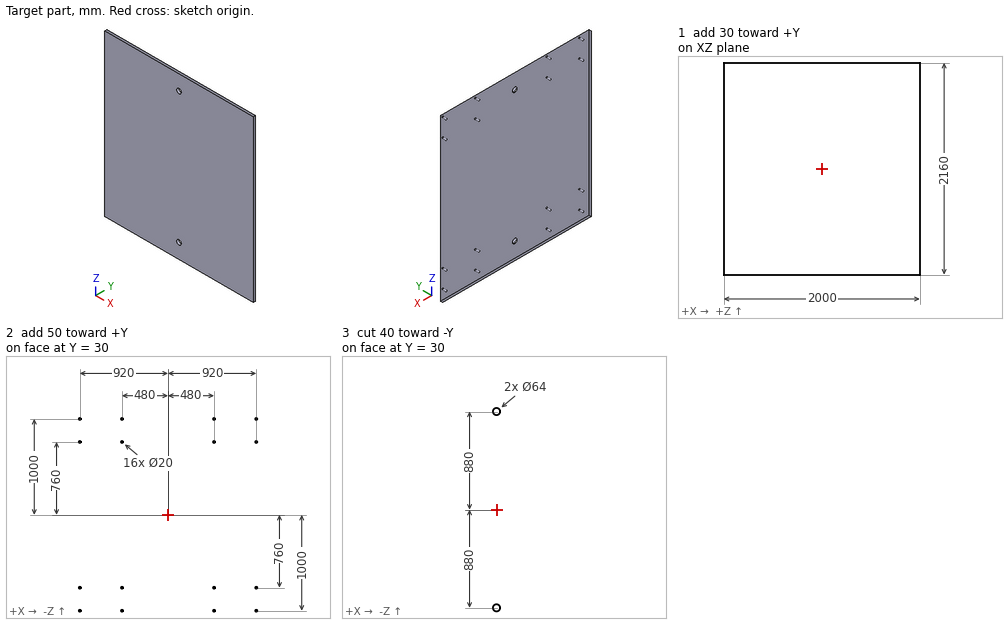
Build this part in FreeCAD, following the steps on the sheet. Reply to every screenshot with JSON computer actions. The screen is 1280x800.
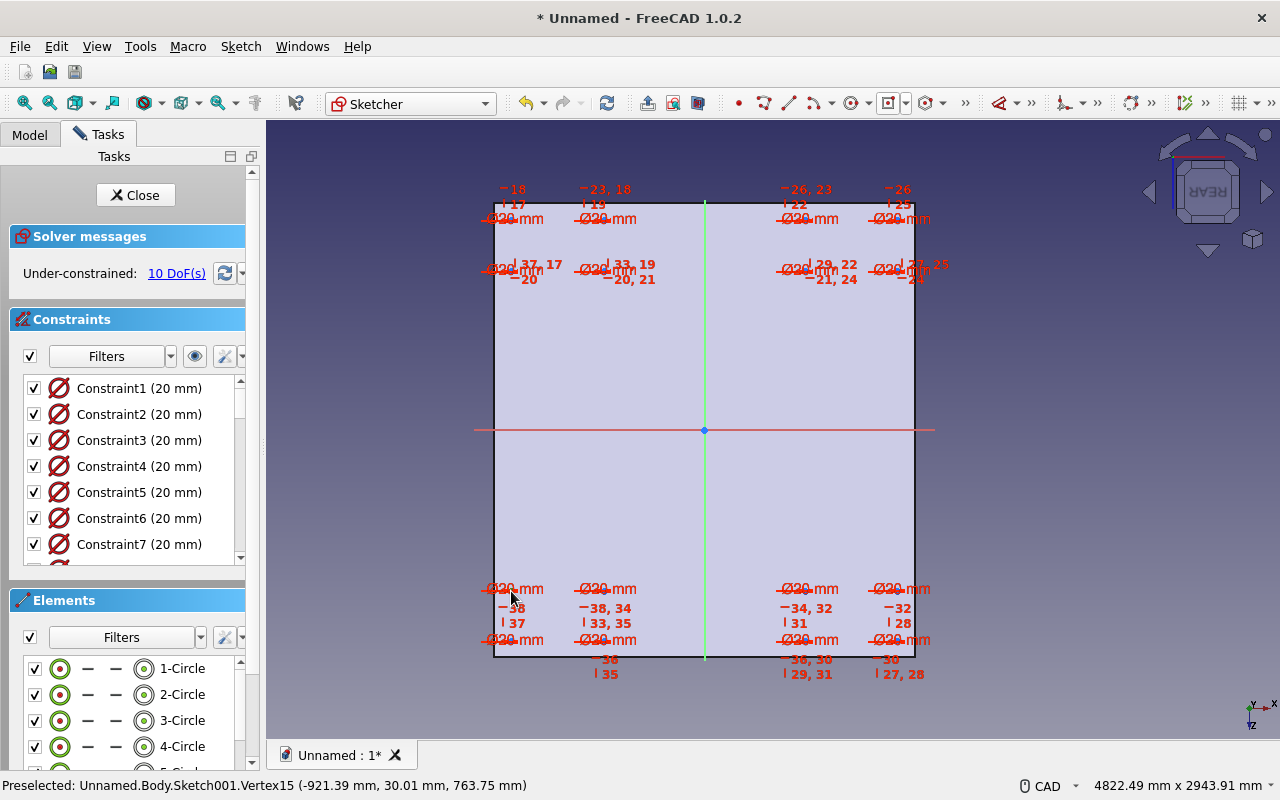
{"action": "left_click", "coordinate": [511, 642]}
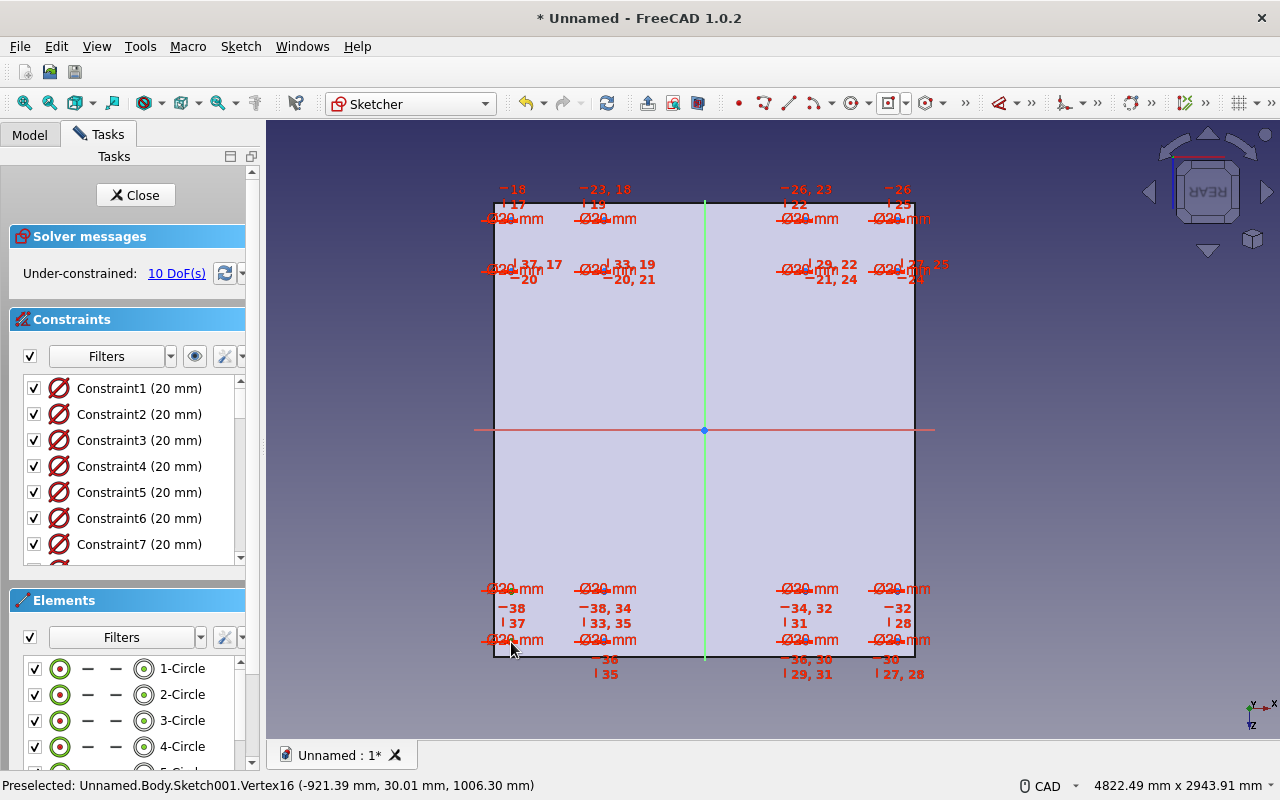
{"action": "key", "text": "v"}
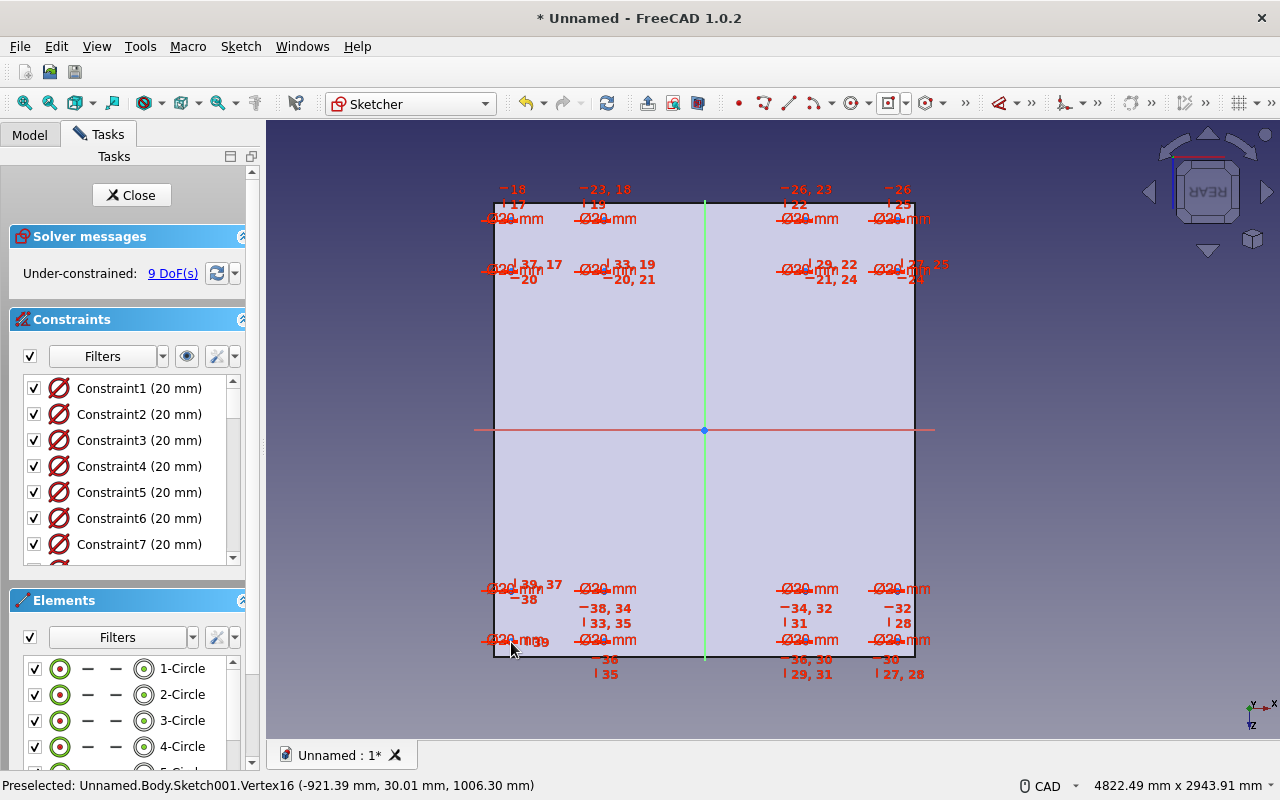
{"action": "left_click", "coordinate": [604, 642]}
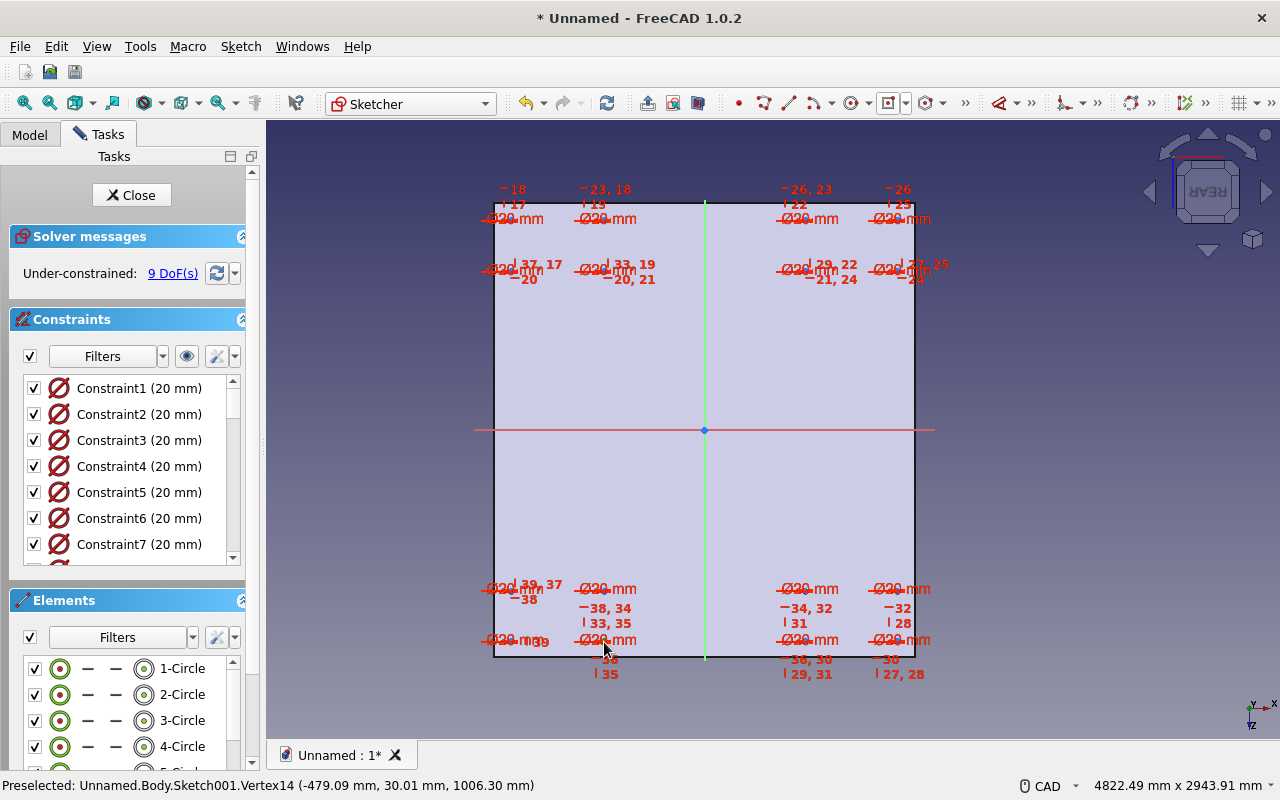
{"action": "left_click", "coordinate": [511, 642]}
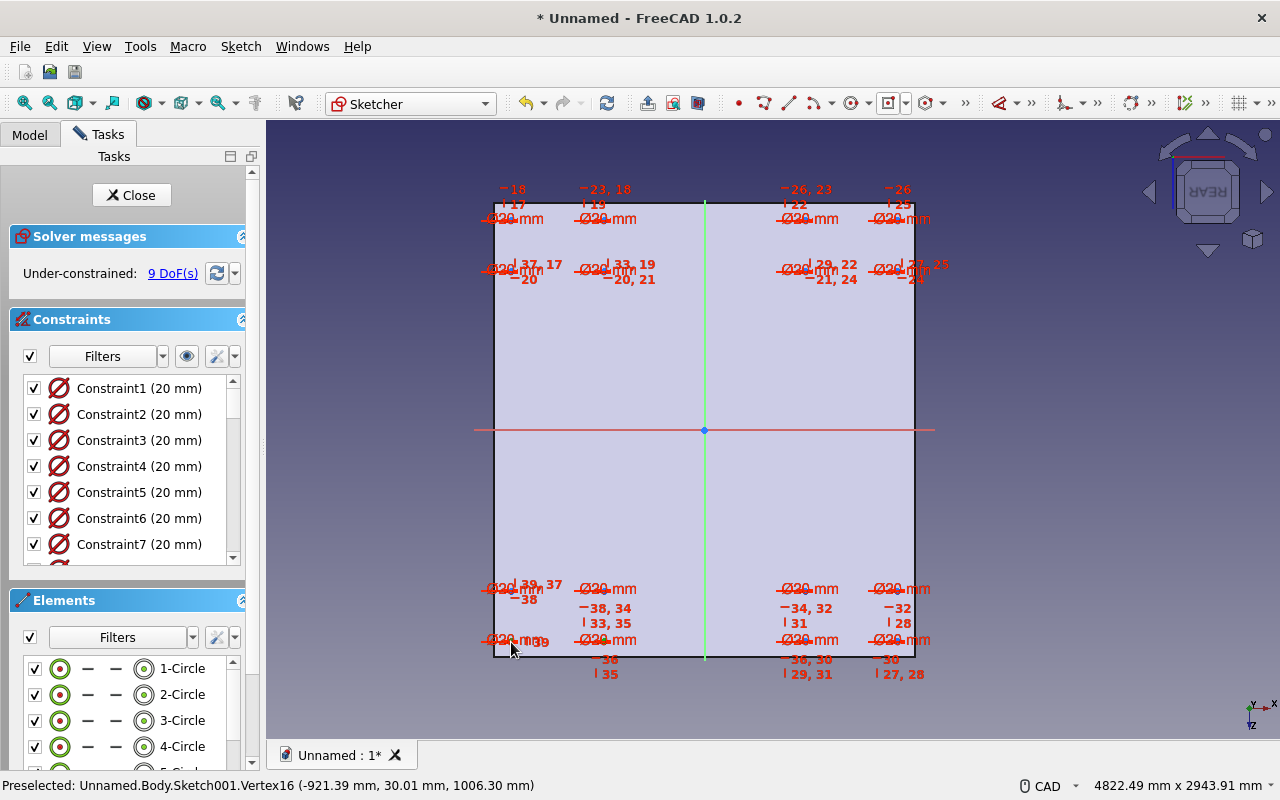
{"action": "key", "text": "h"}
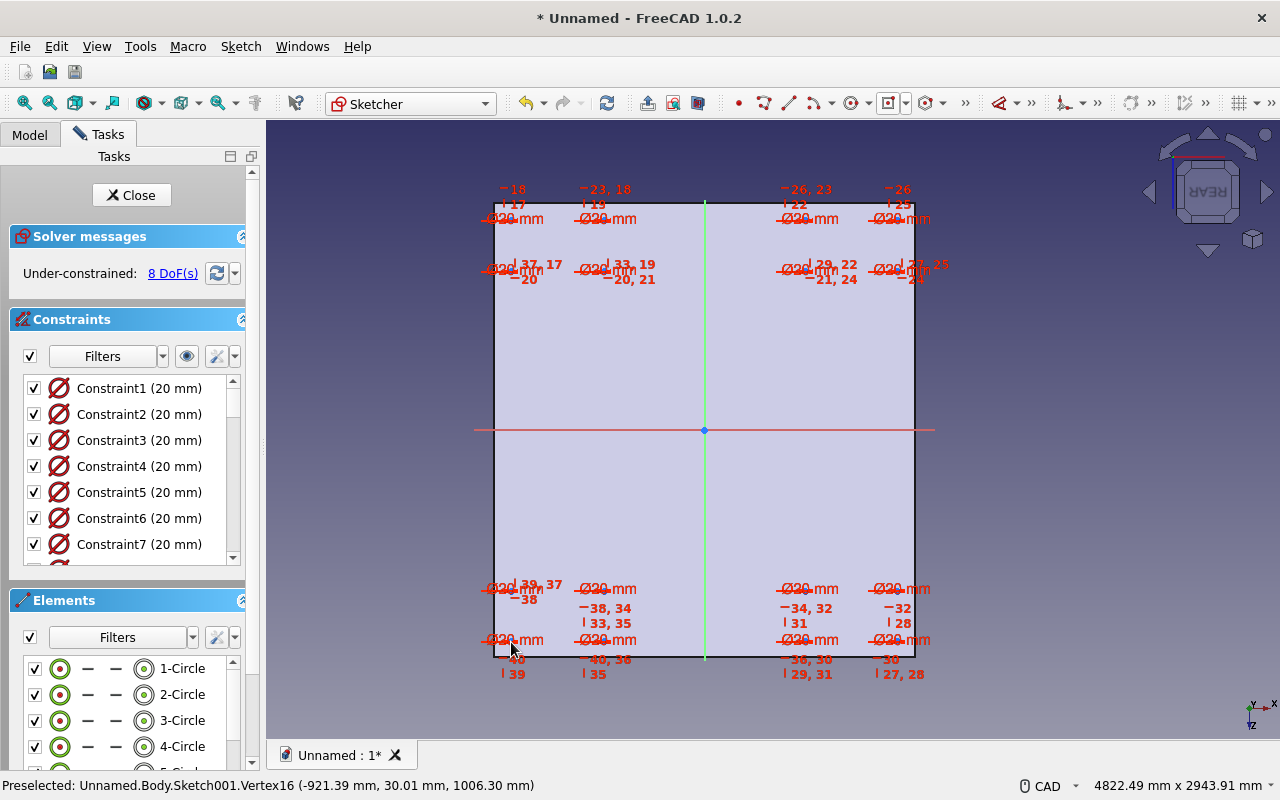
{"action": "left_click", "coordinate": [998, 104]}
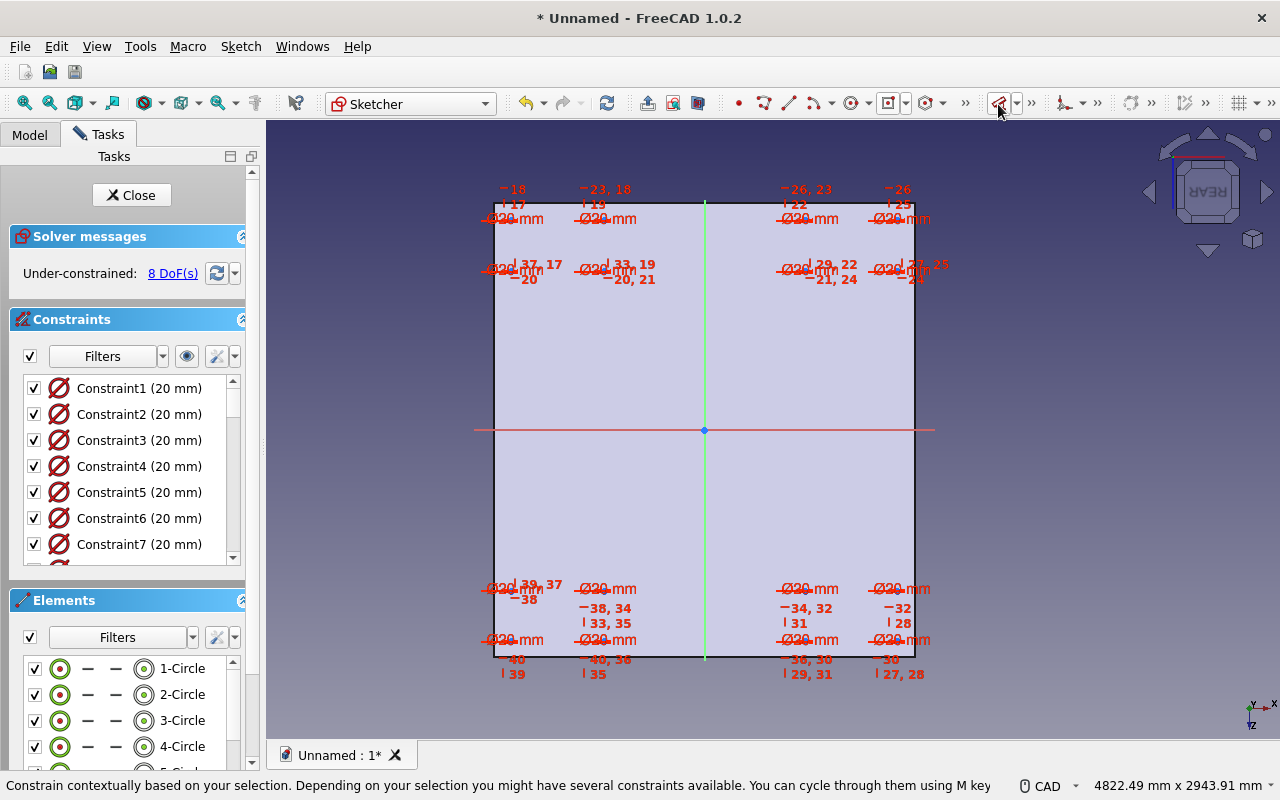
{"action": "left_click", "coordinate": [511, 221]}
{"action": "left_click", "coordinate": [608, 187]}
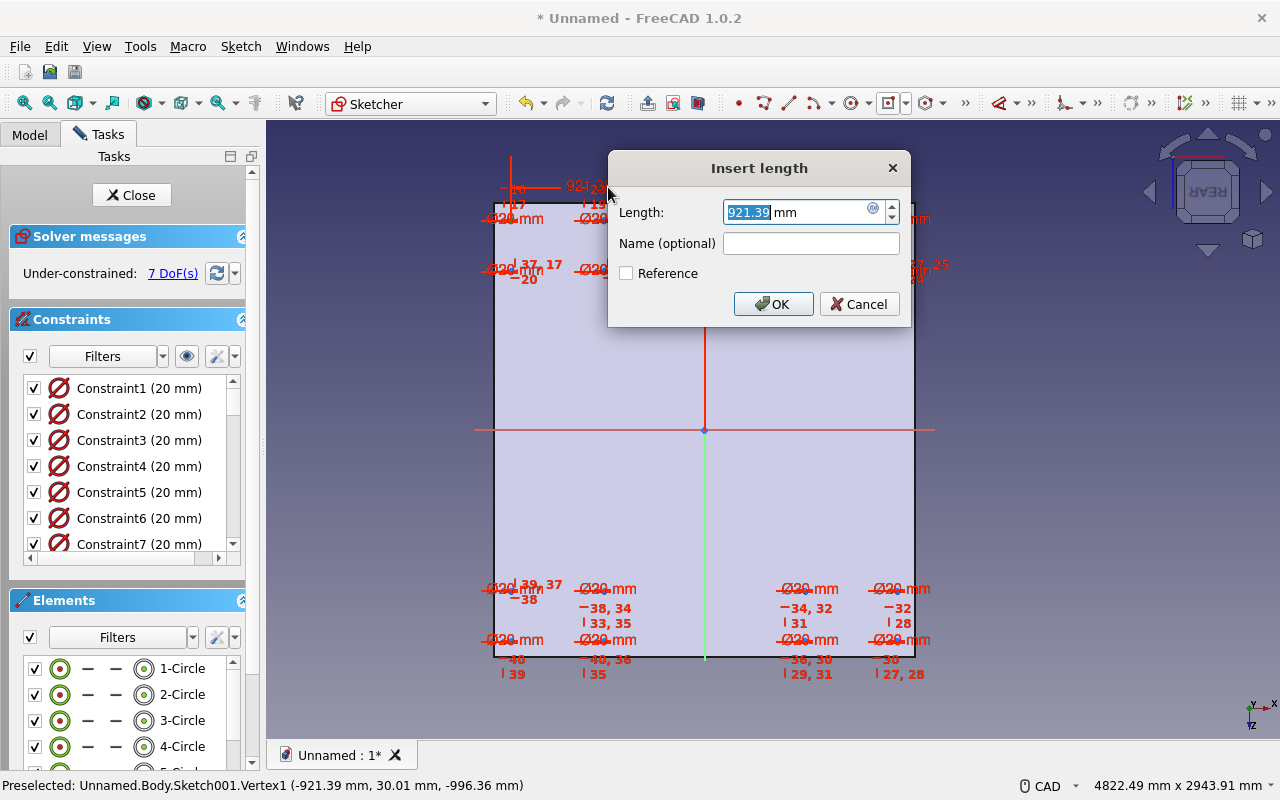
{"action": "type", "text": "920"}
{"action": "key", "text": "Return"}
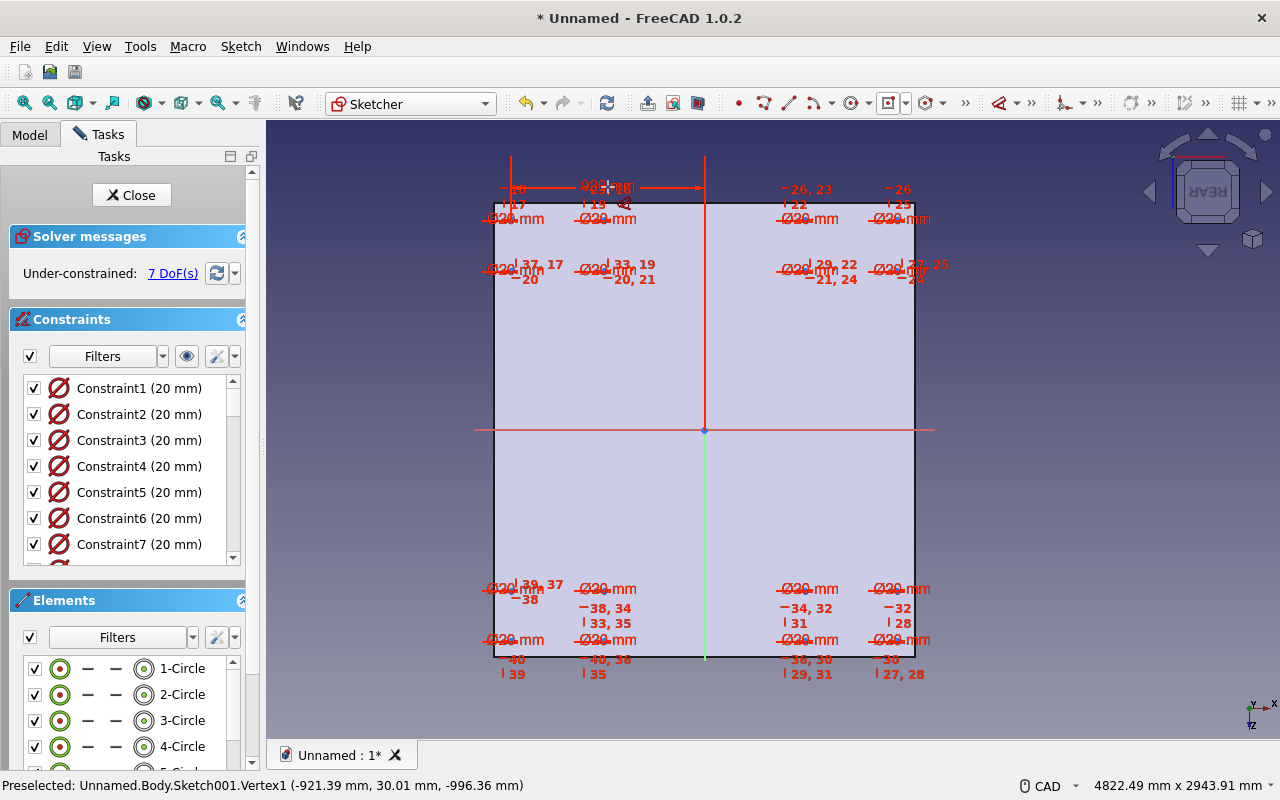
{"action": "left_click", "coordinate": [511, 272]}
{"action": "left_click", "coordinate": [477, 351]}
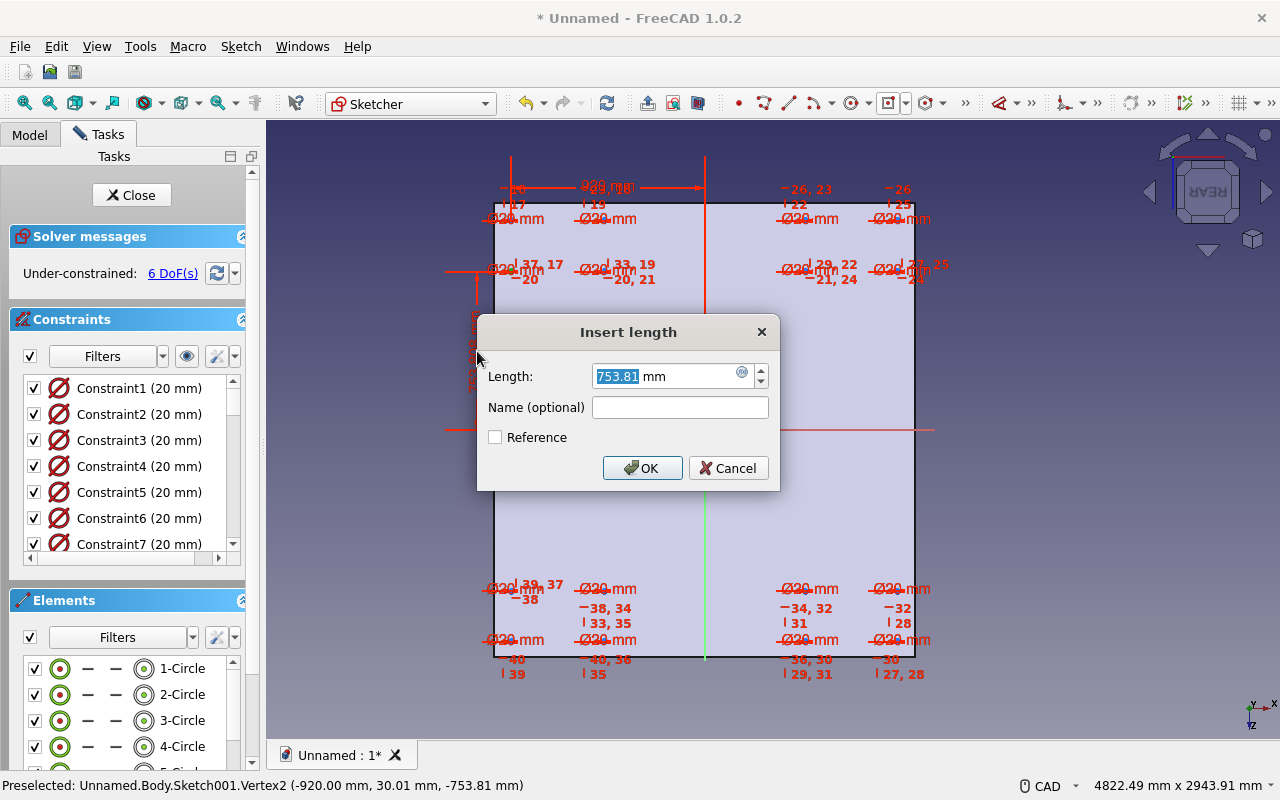
{"action": "type", "text": "760"}
{"action": "key", "text": "Return"}